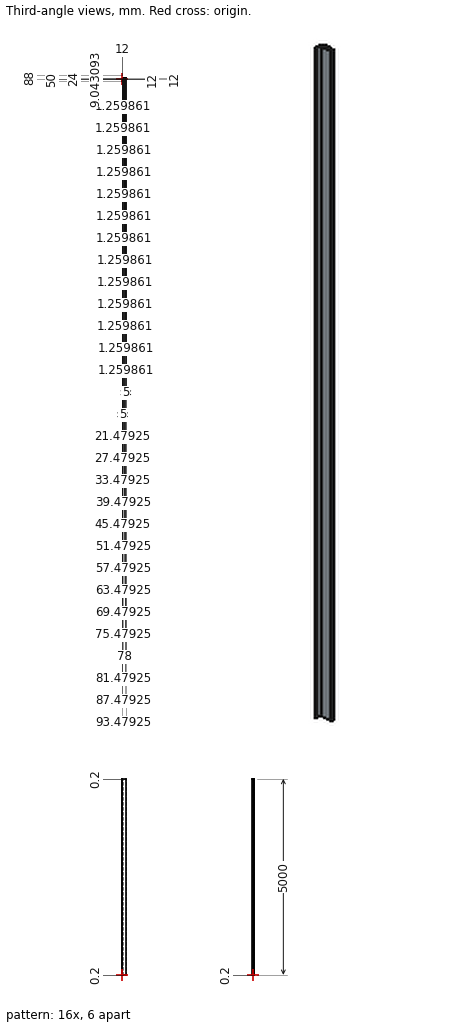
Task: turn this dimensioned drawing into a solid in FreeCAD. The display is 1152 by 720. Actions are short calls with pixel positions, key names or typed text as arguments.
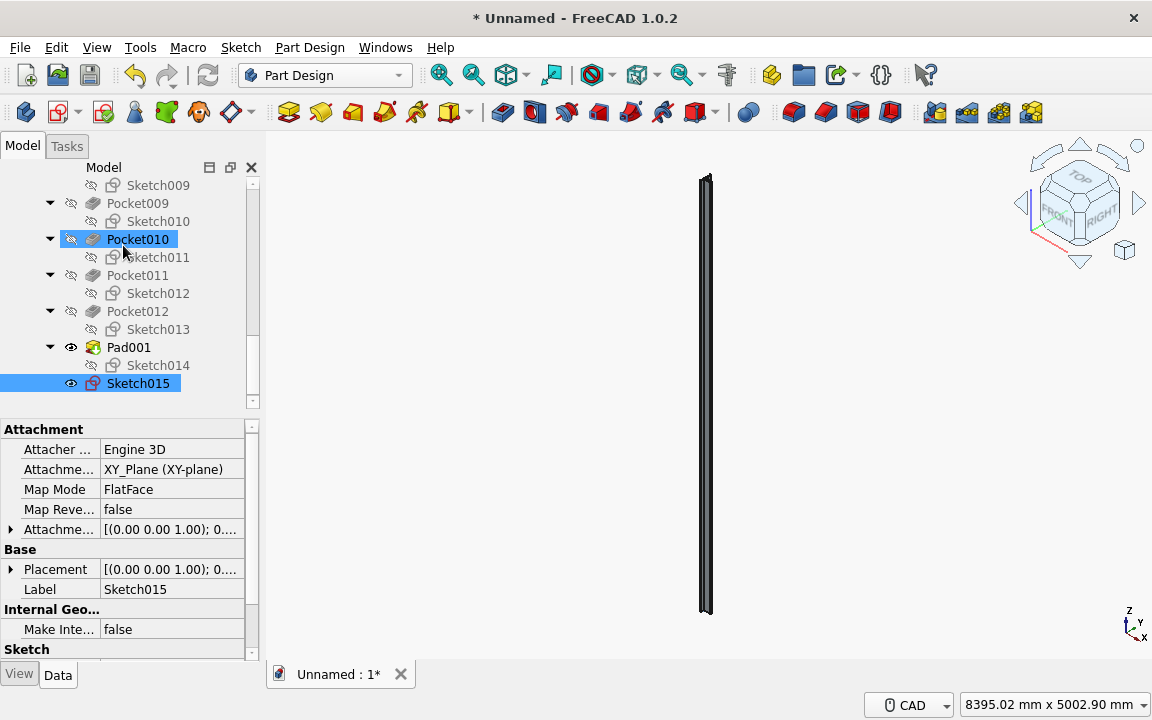
click(504, 112)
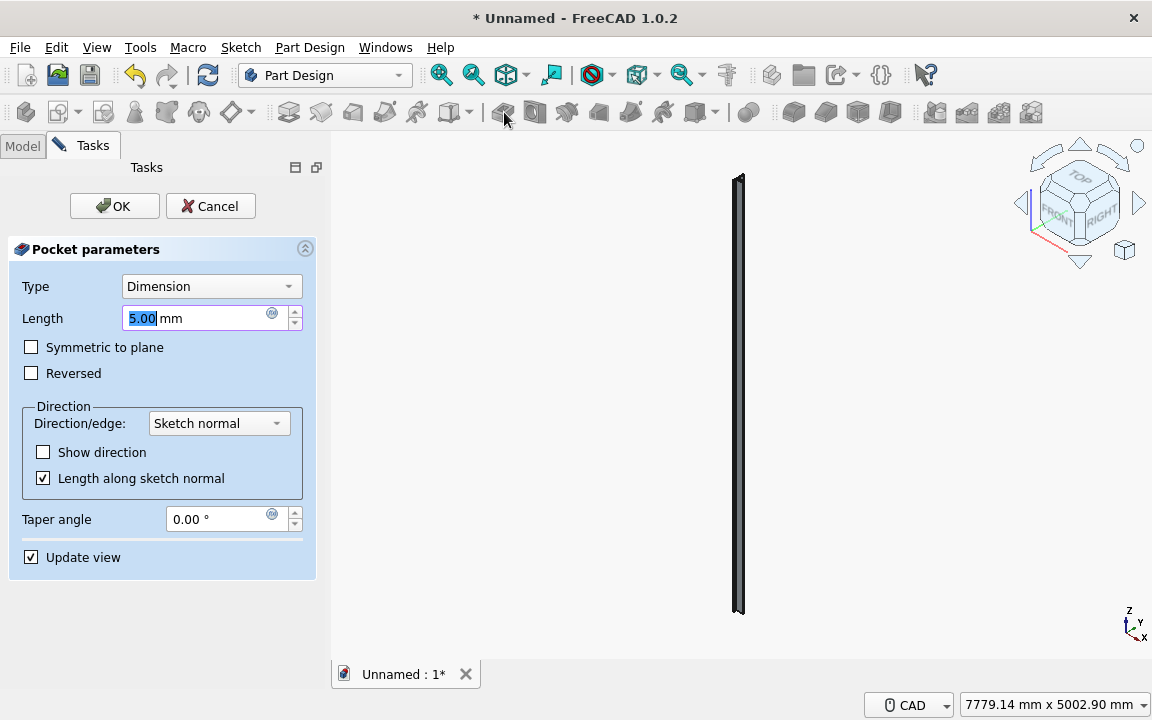
click(212, 286)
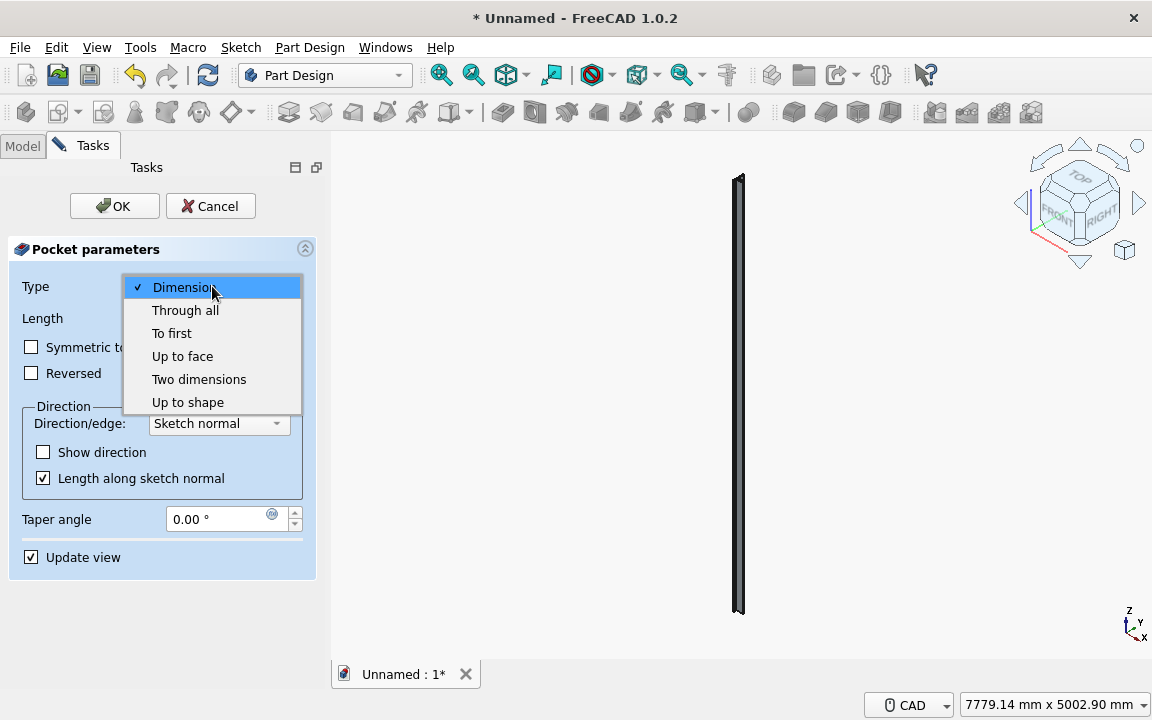
click(212, 310)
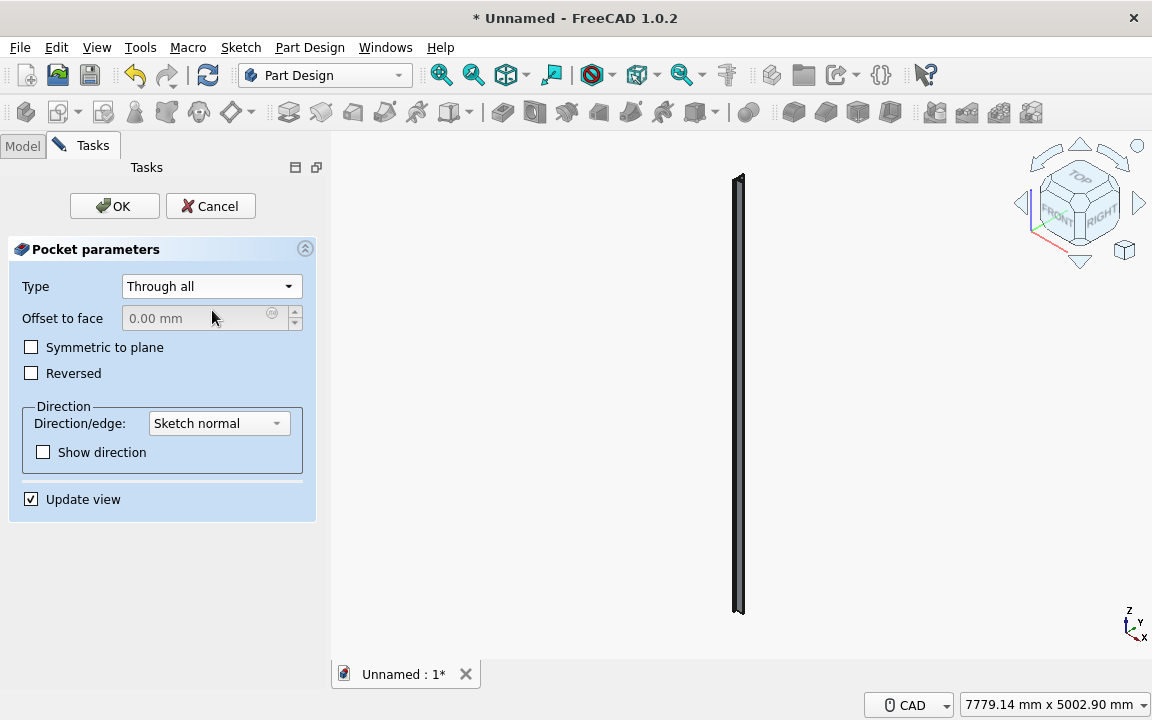
click(30, 373)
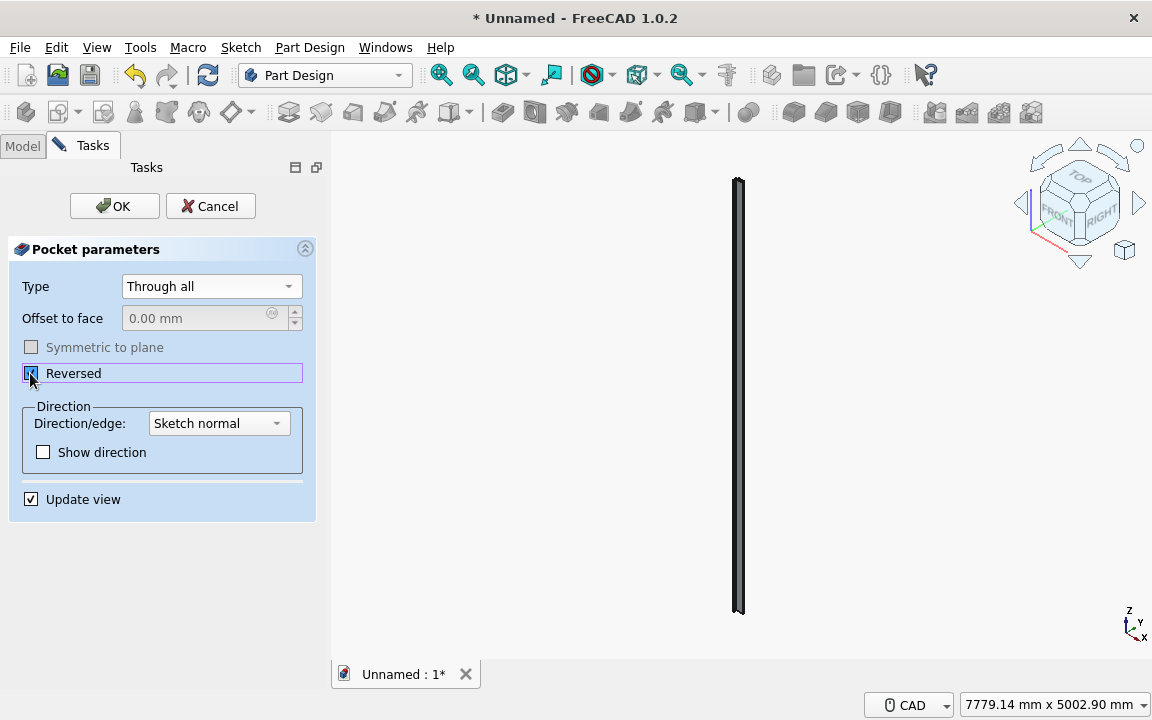
click(115, 206)